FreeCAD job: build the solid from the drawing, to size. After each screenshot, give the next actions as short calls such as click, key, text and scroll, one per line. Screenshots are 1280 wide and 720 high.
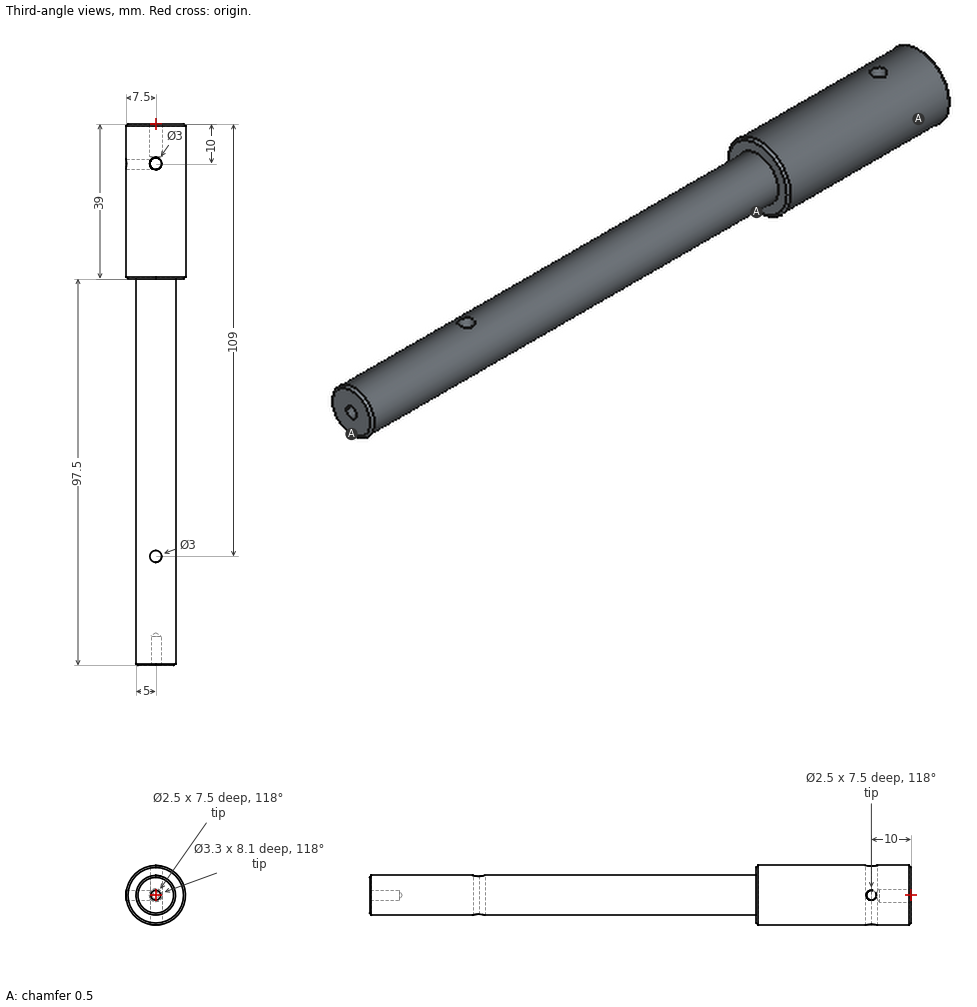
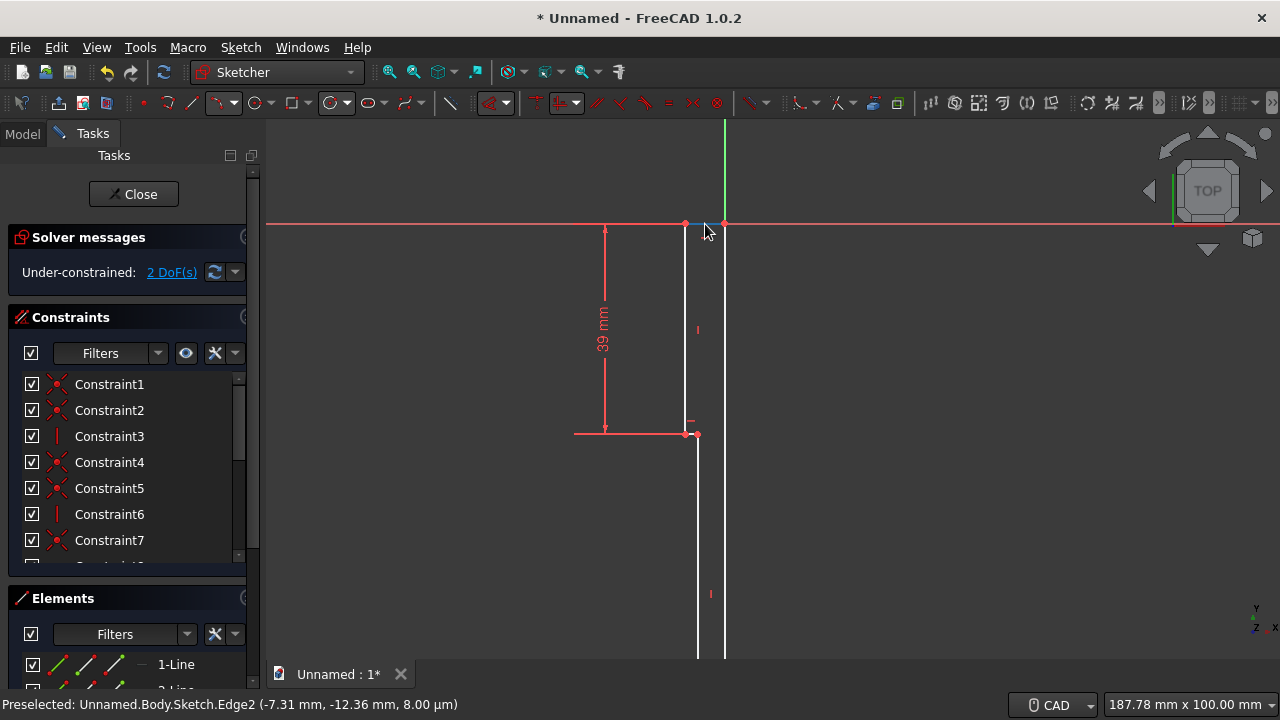
click(705, 224)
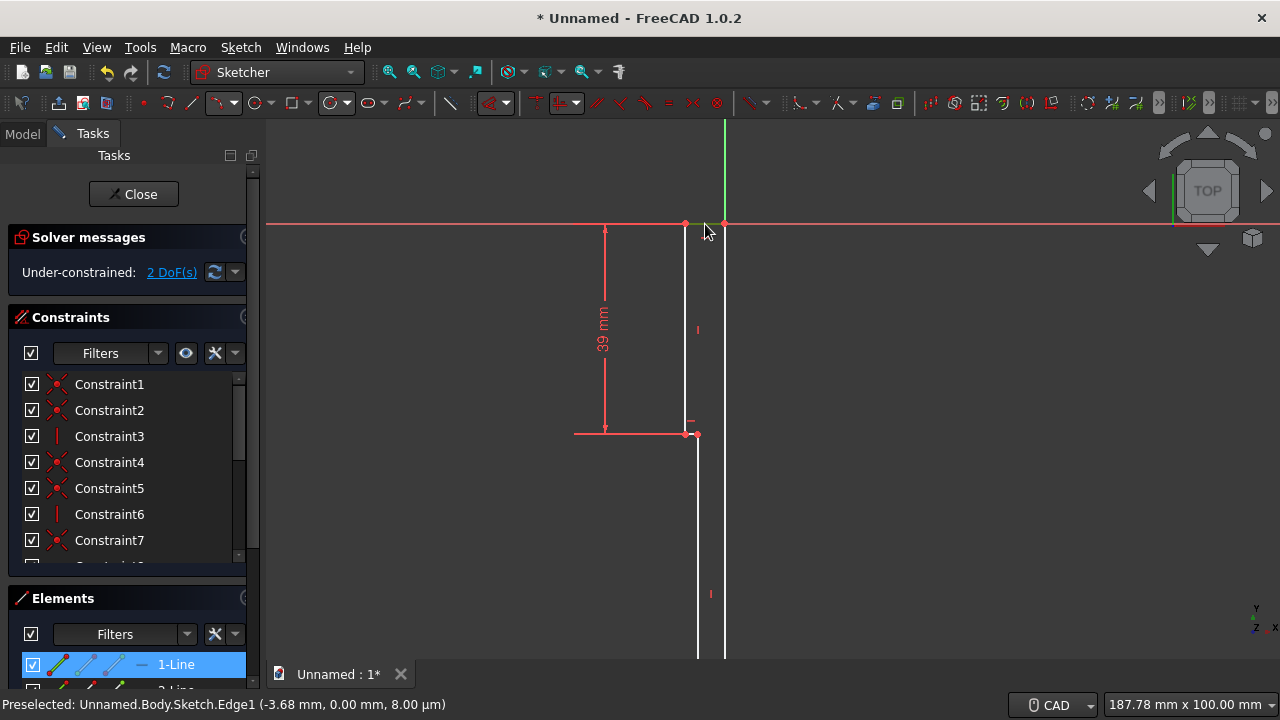
click(508, 104)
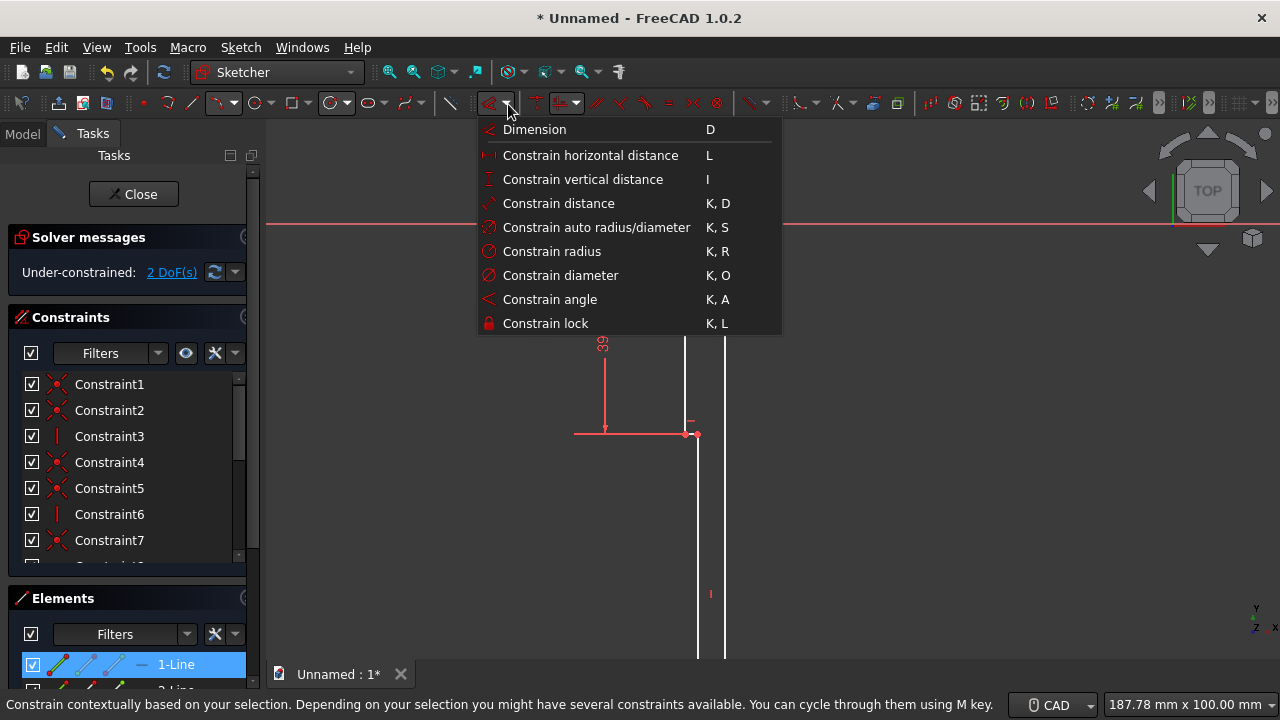
click(630, 155)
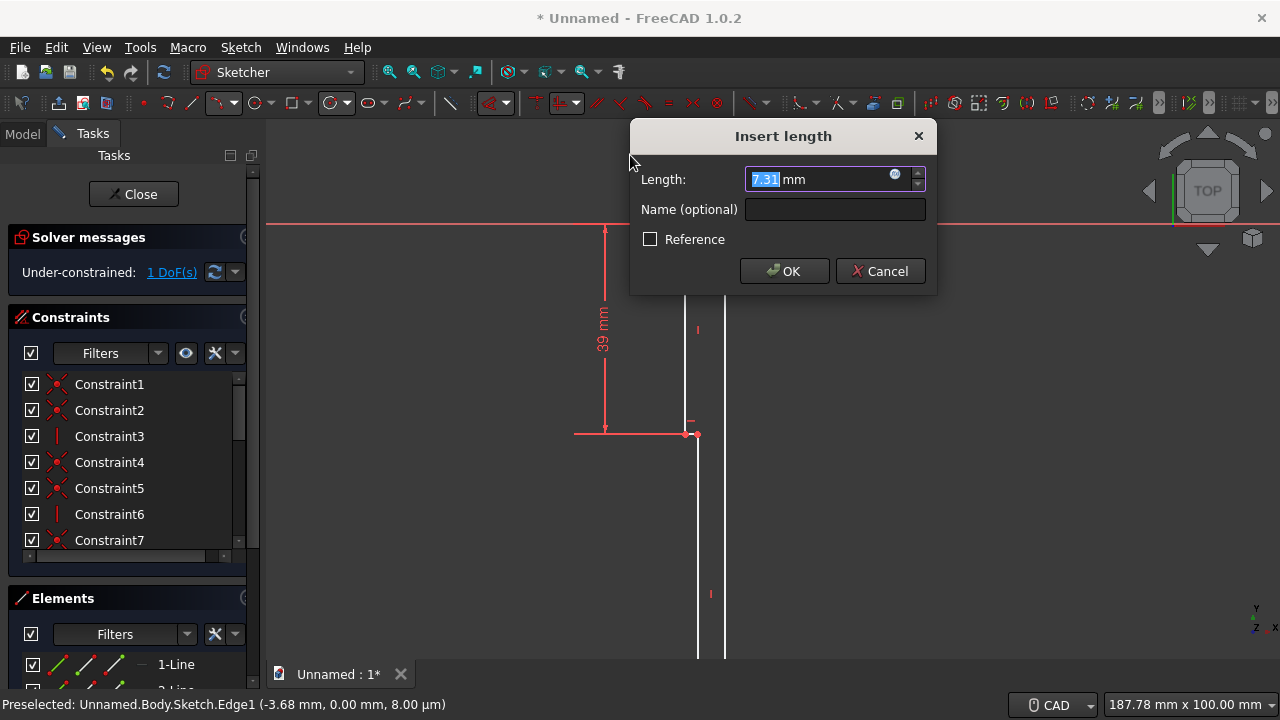
text(7.5)
key(Return)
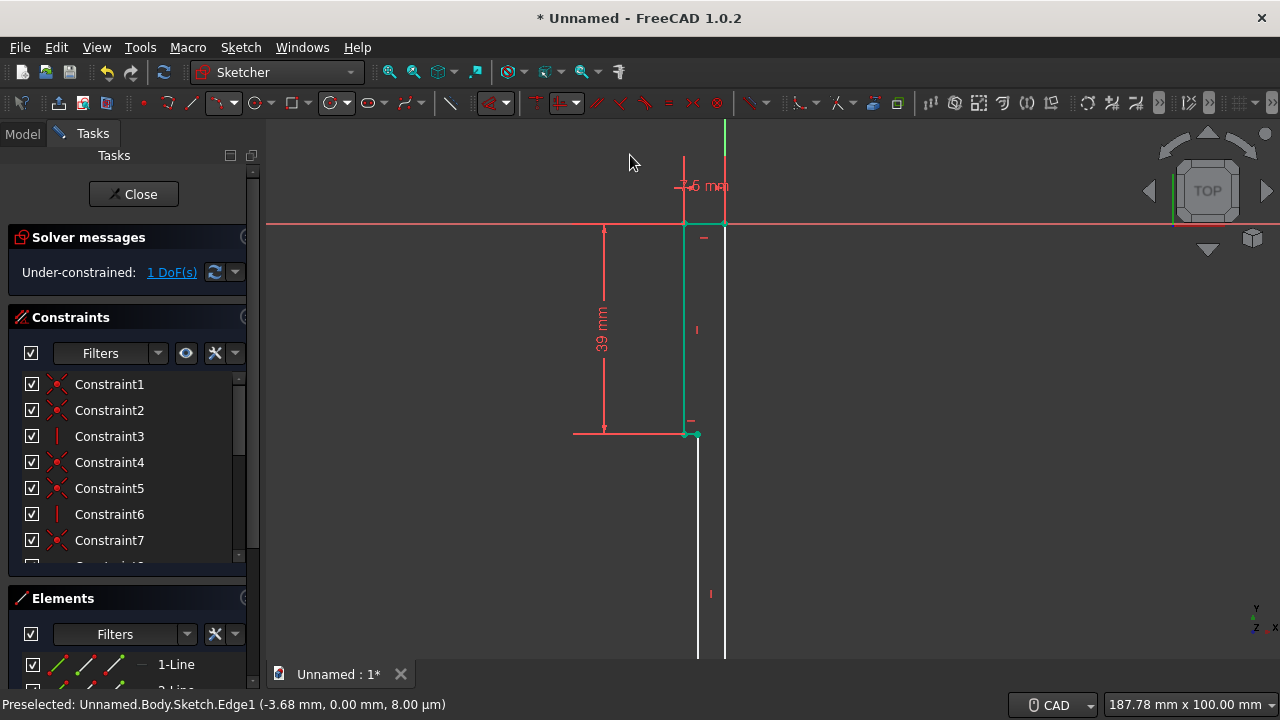
click(698, 593)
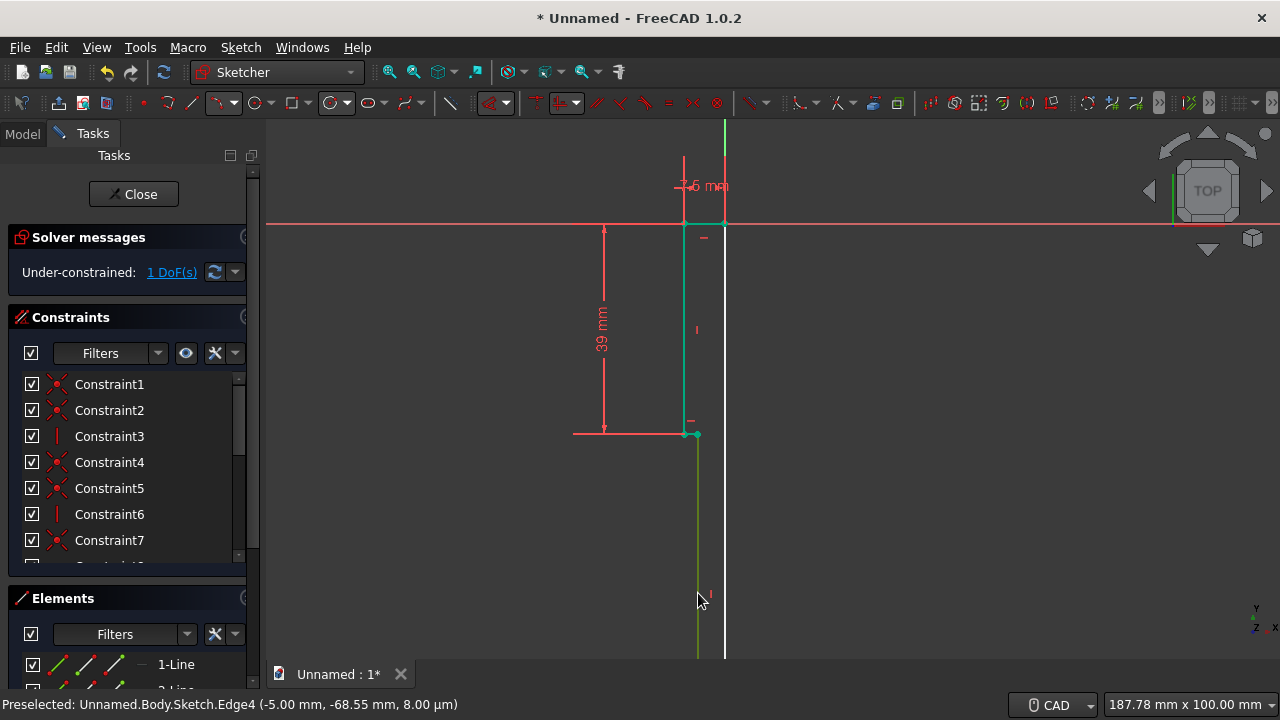
click(508, 104)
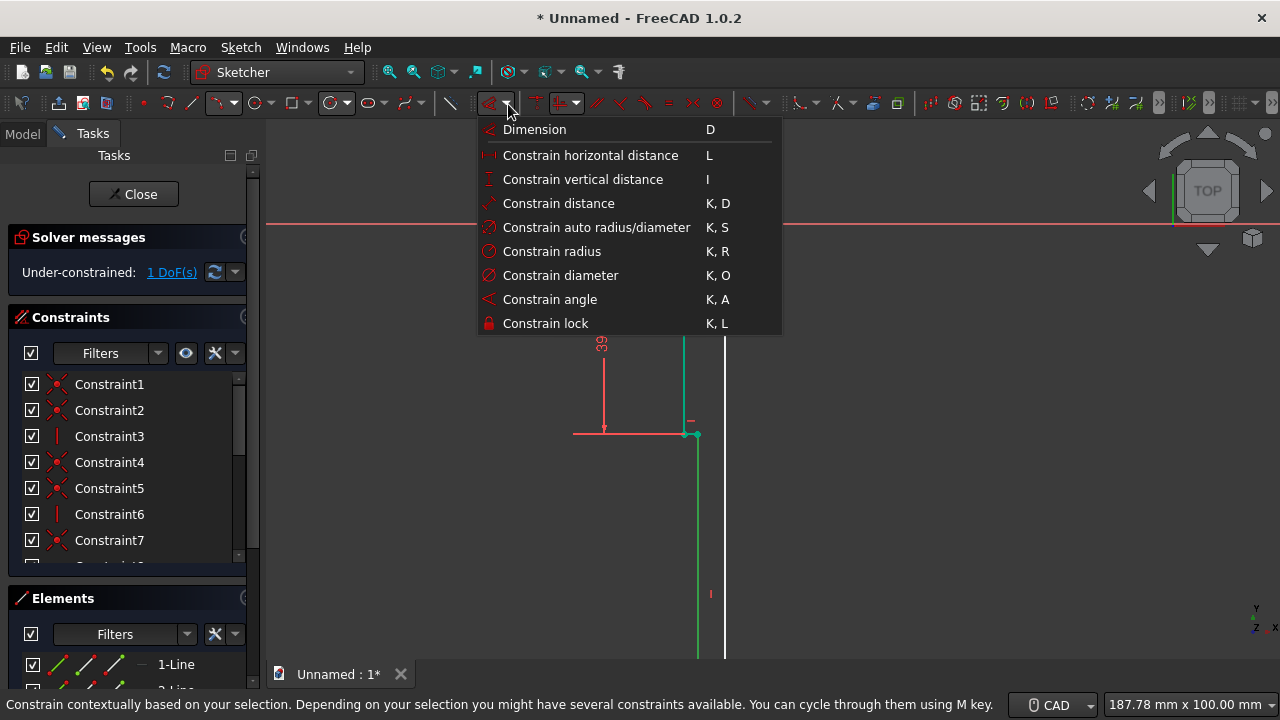
click(630, 179)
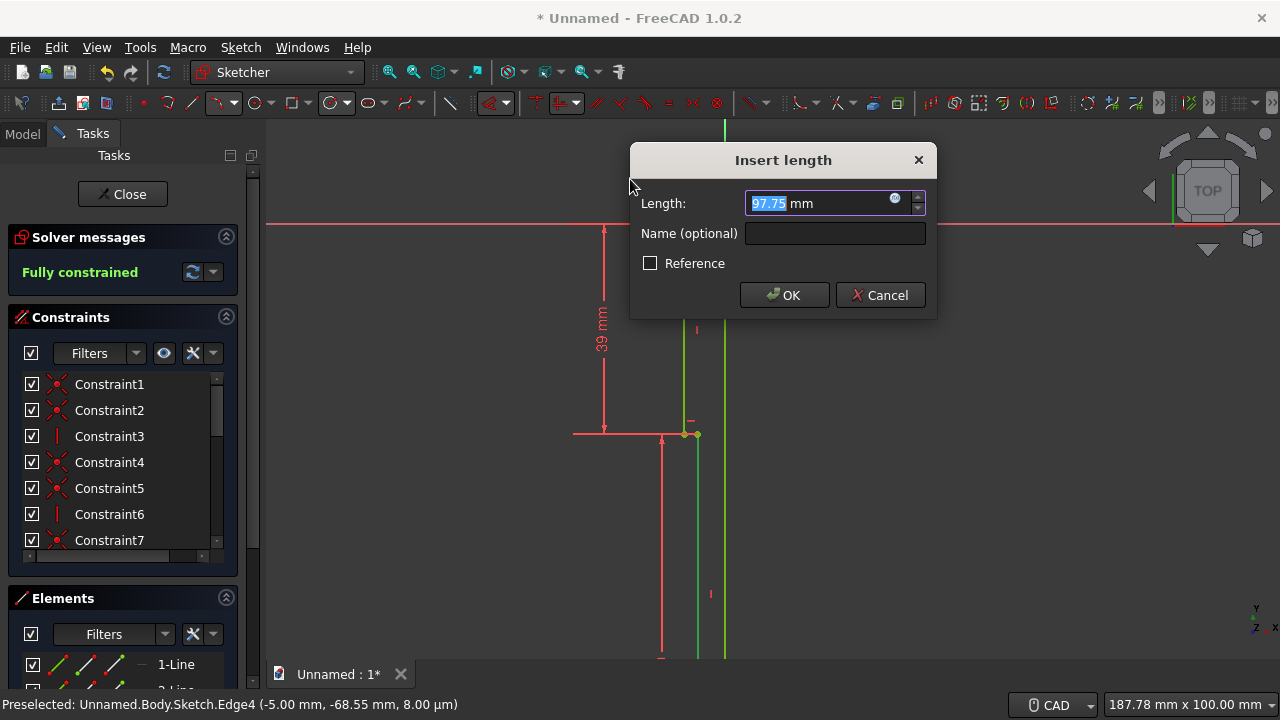
text(97.5)
key(Return)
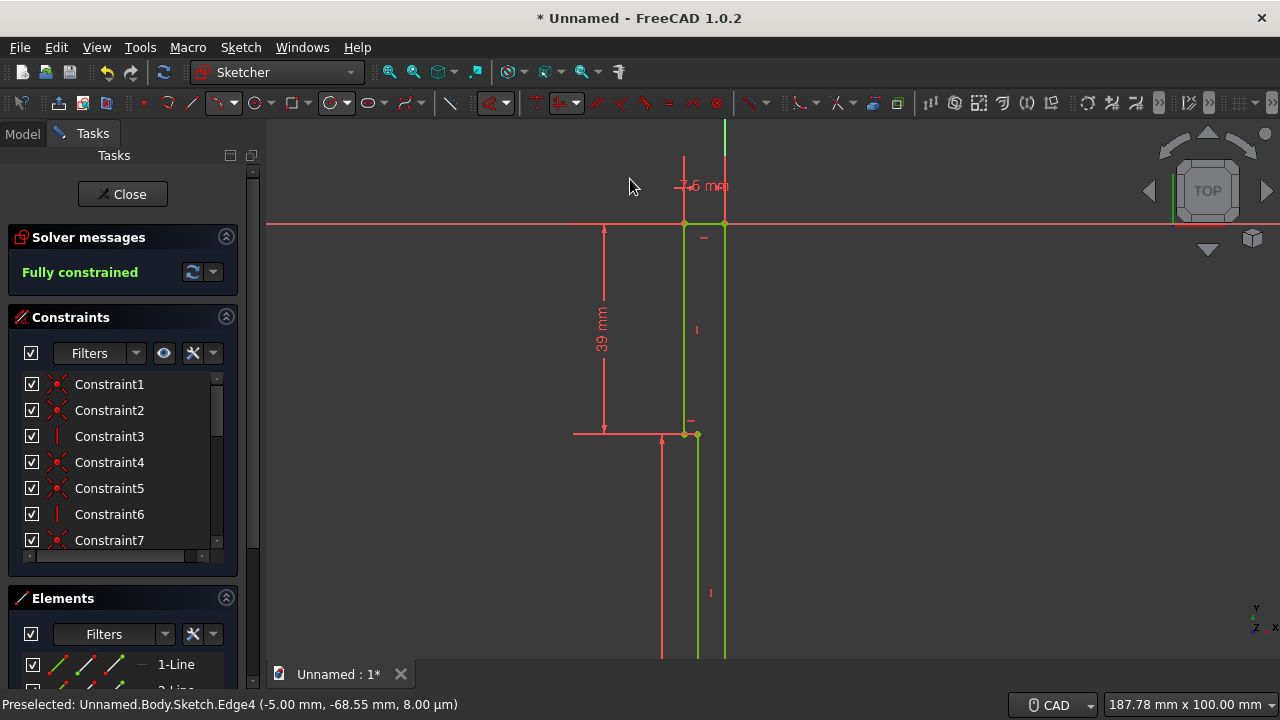
click(123, 194)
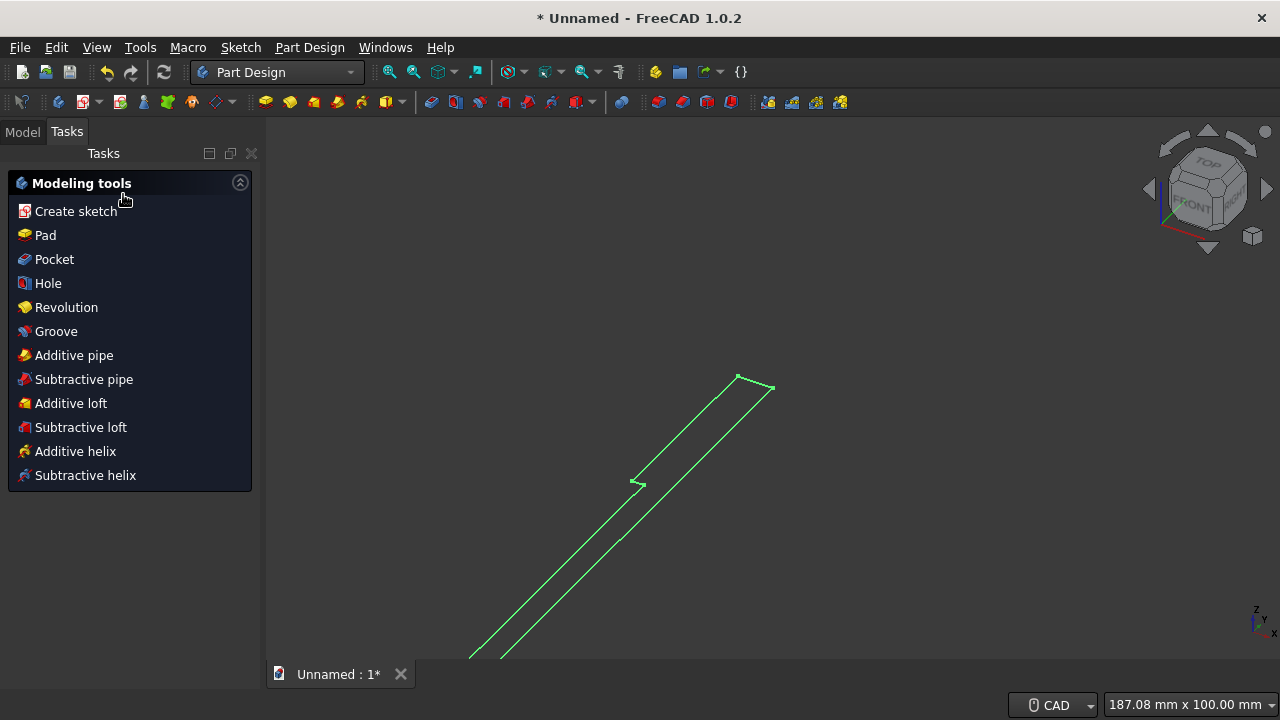
click(290, 102)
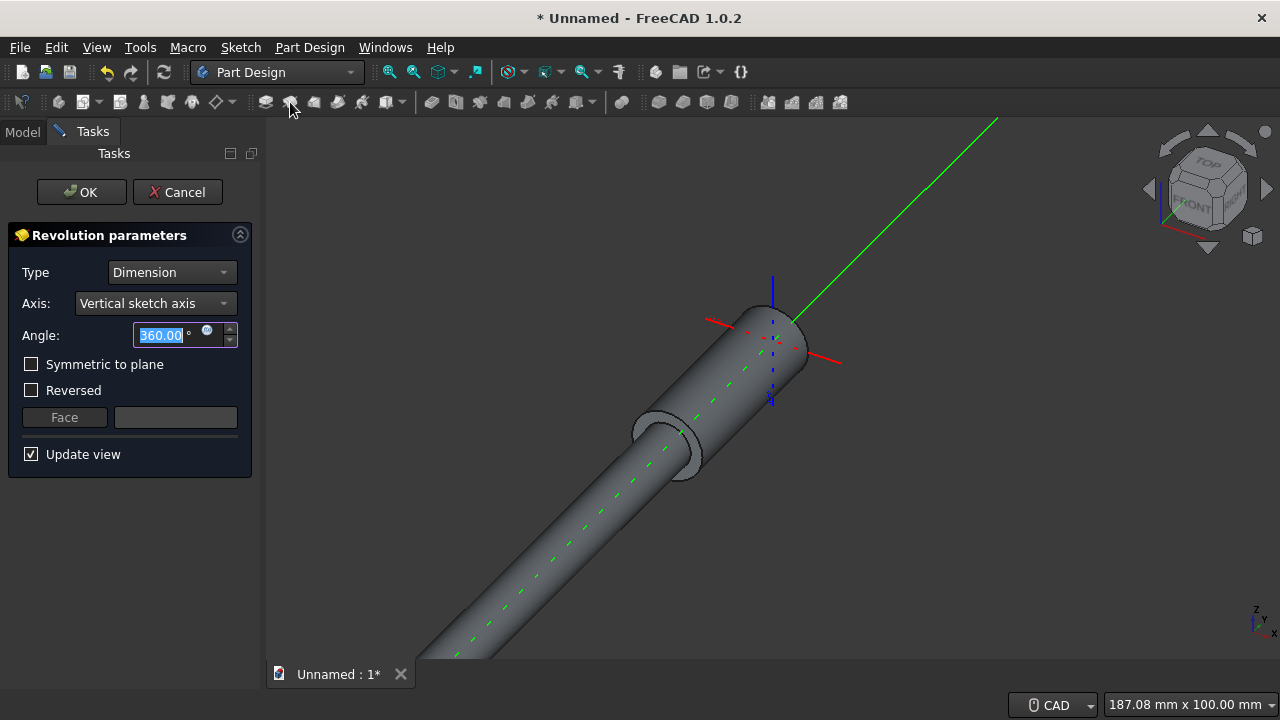
click(82, 192)